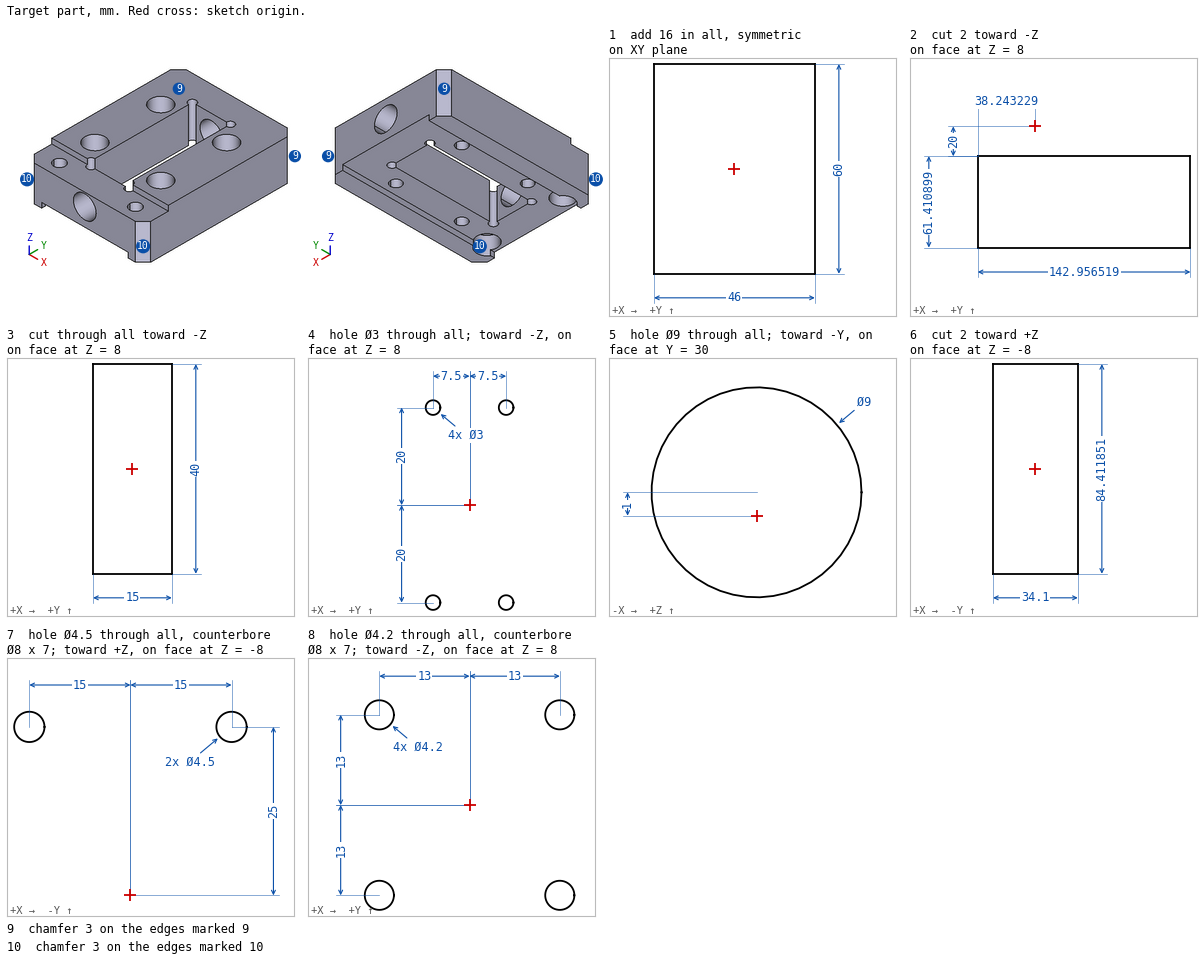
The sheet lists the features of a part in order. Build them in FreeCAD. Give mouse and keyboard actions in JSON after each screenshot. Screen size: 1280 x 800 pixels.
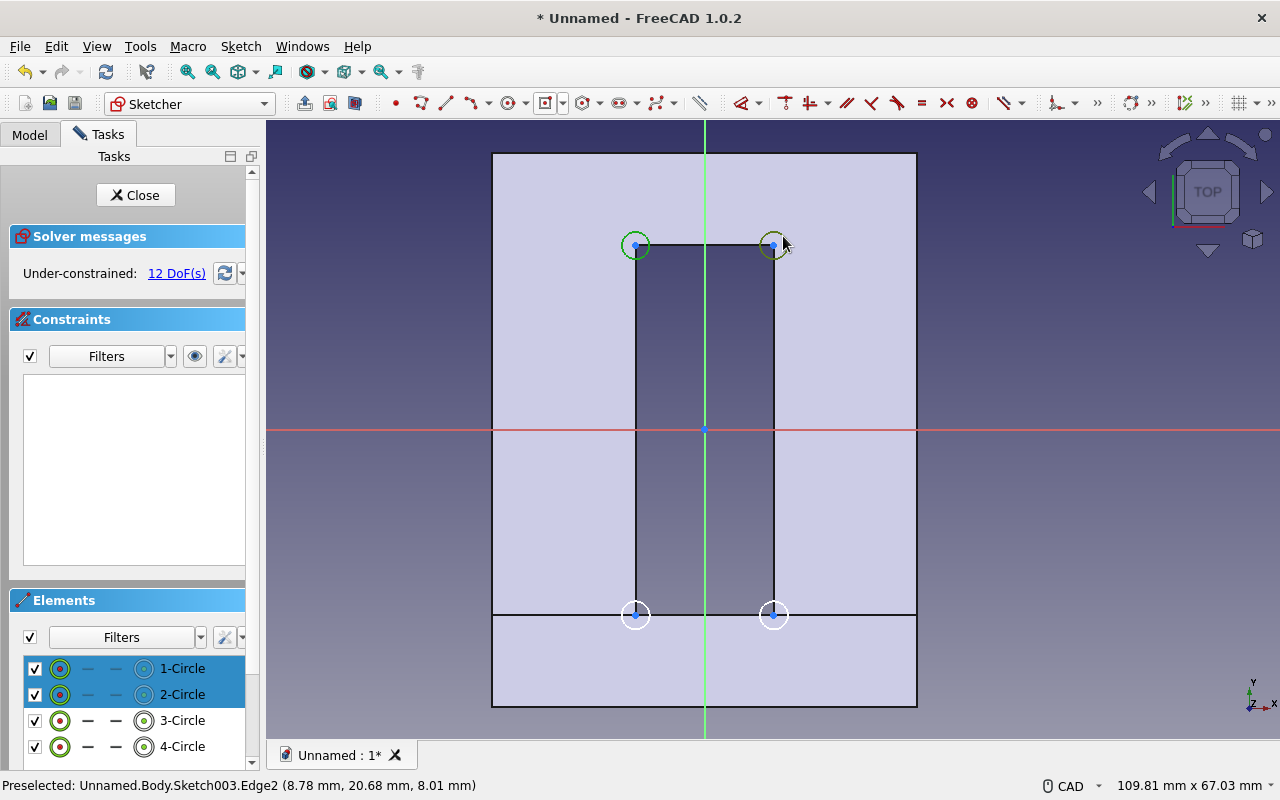
{"action": "left_click", "coordinate": [645, 605]}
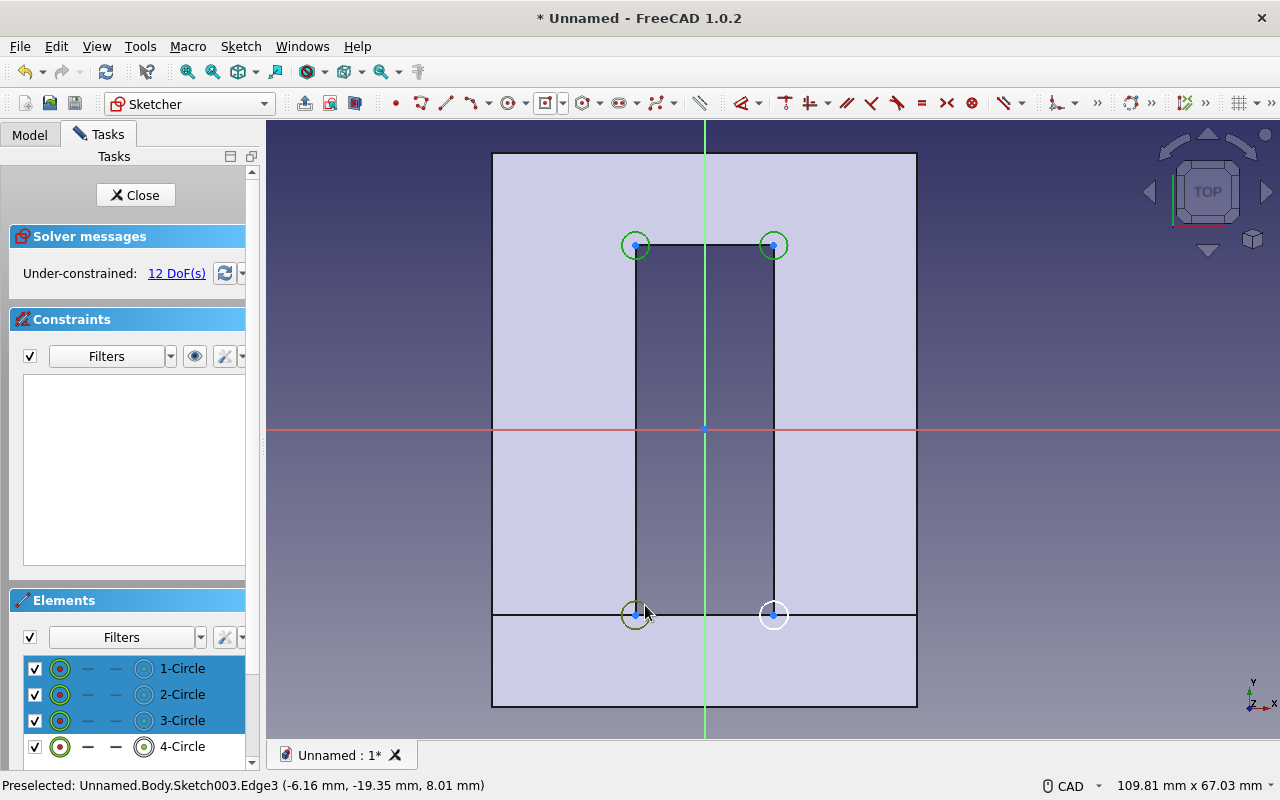
{"action": "left_click", "coordinate": [784, 605]}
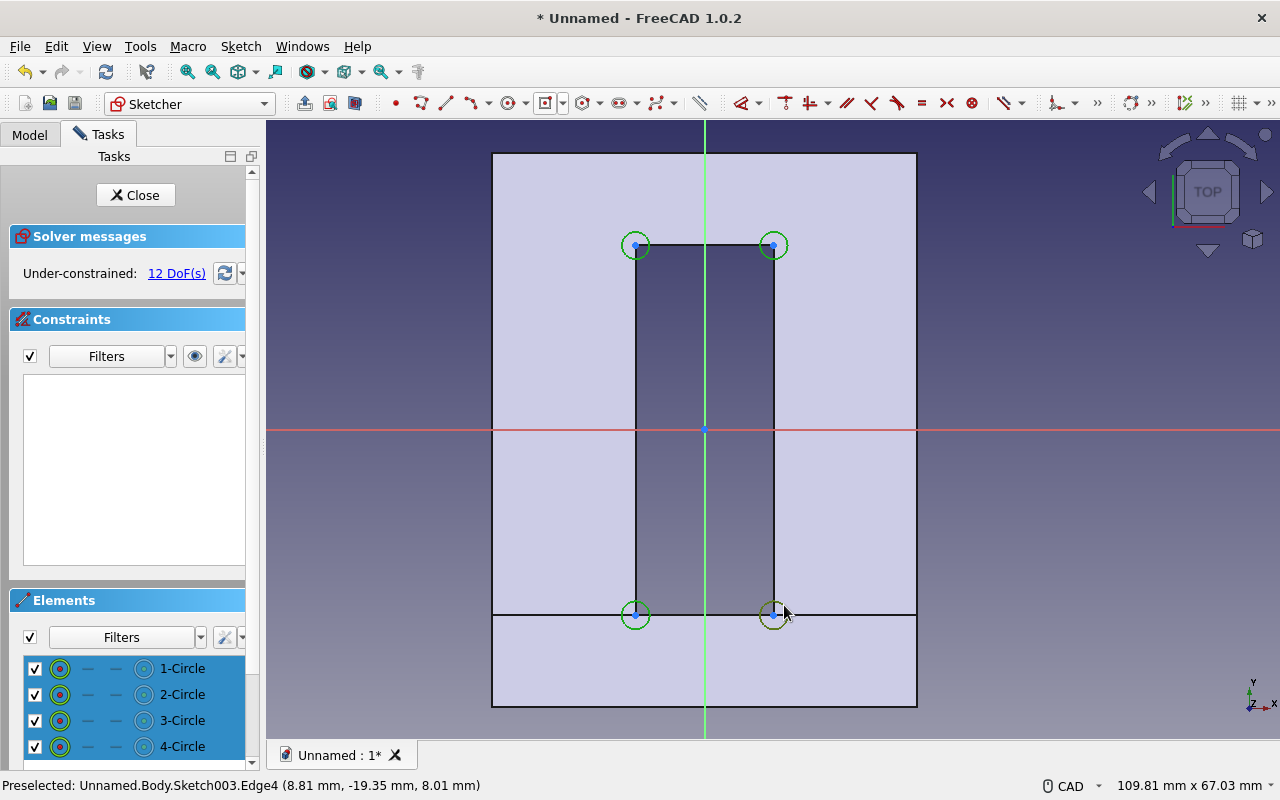
{"action": "left_click", "coordinate": [922, 104]}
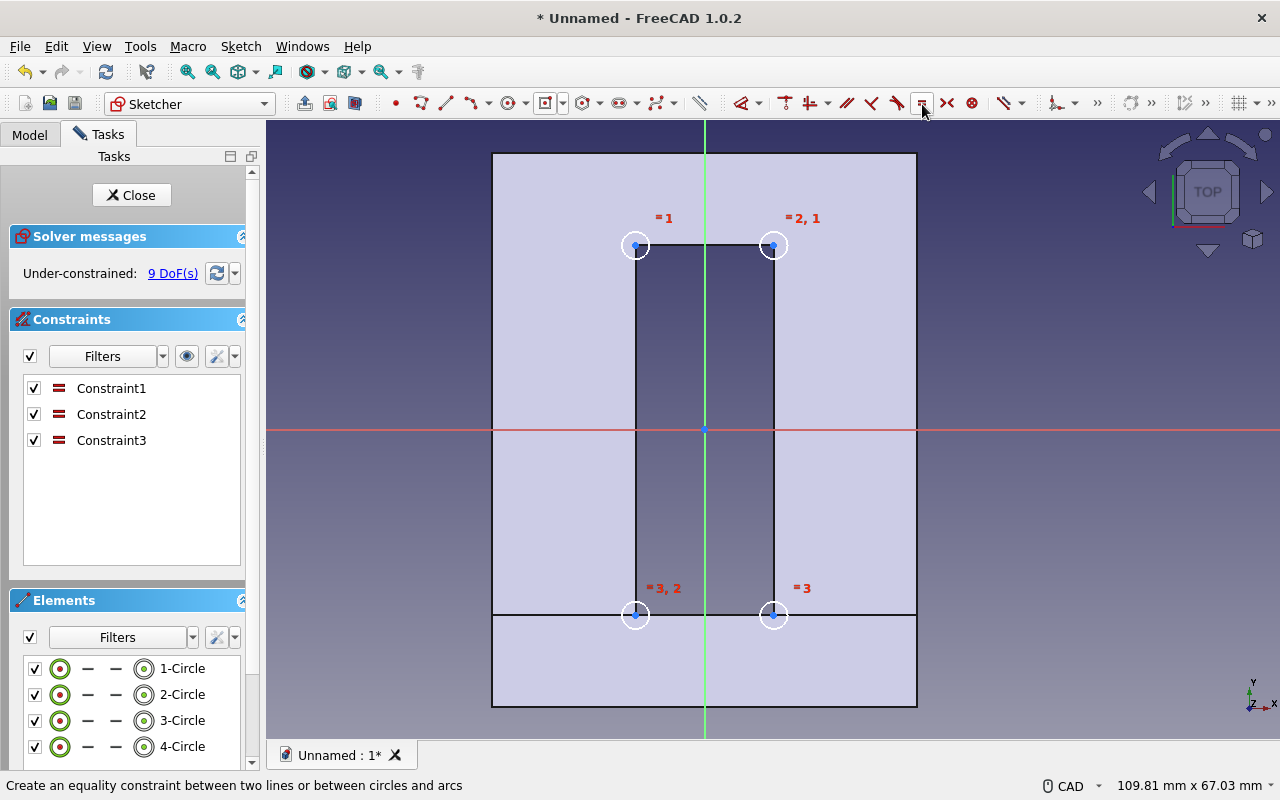
{"action": "left_click", "coordinate": [636, 246]}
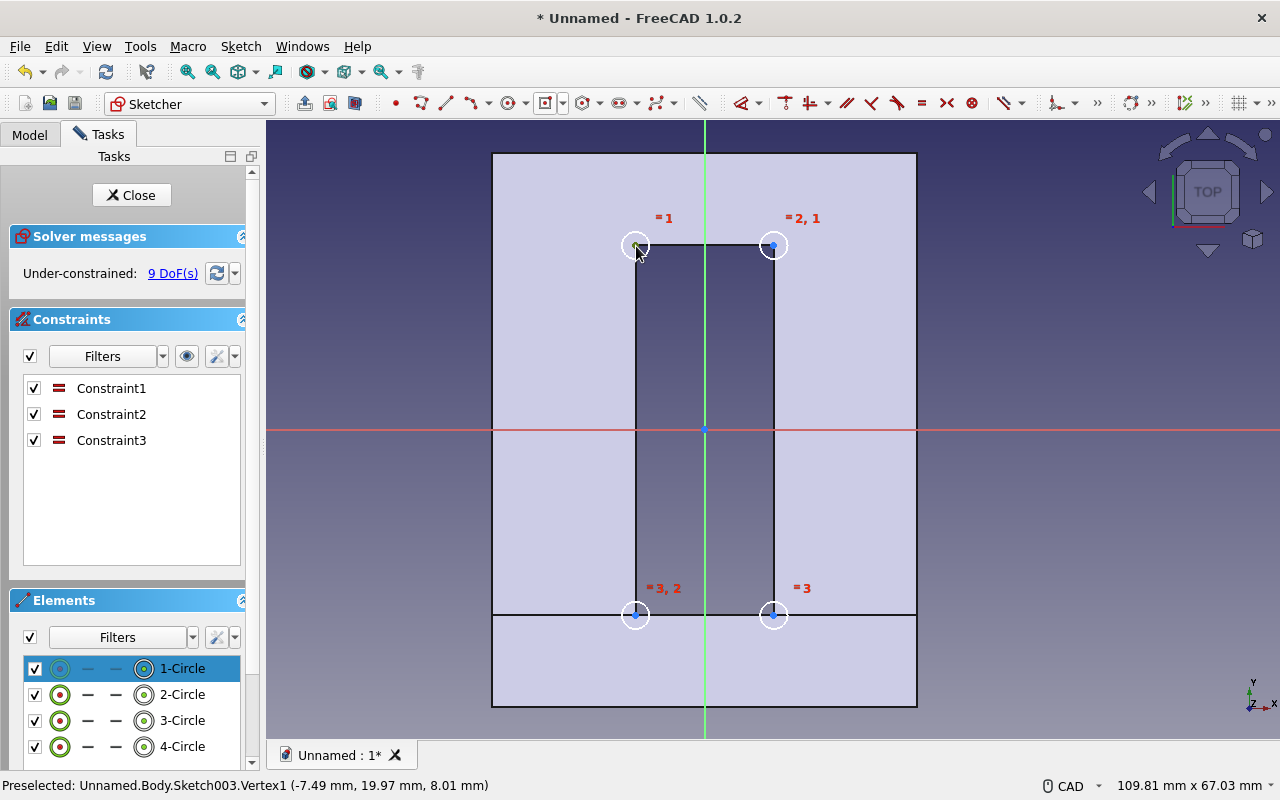
{"action": "left_click", "coordinate": [774, 246]}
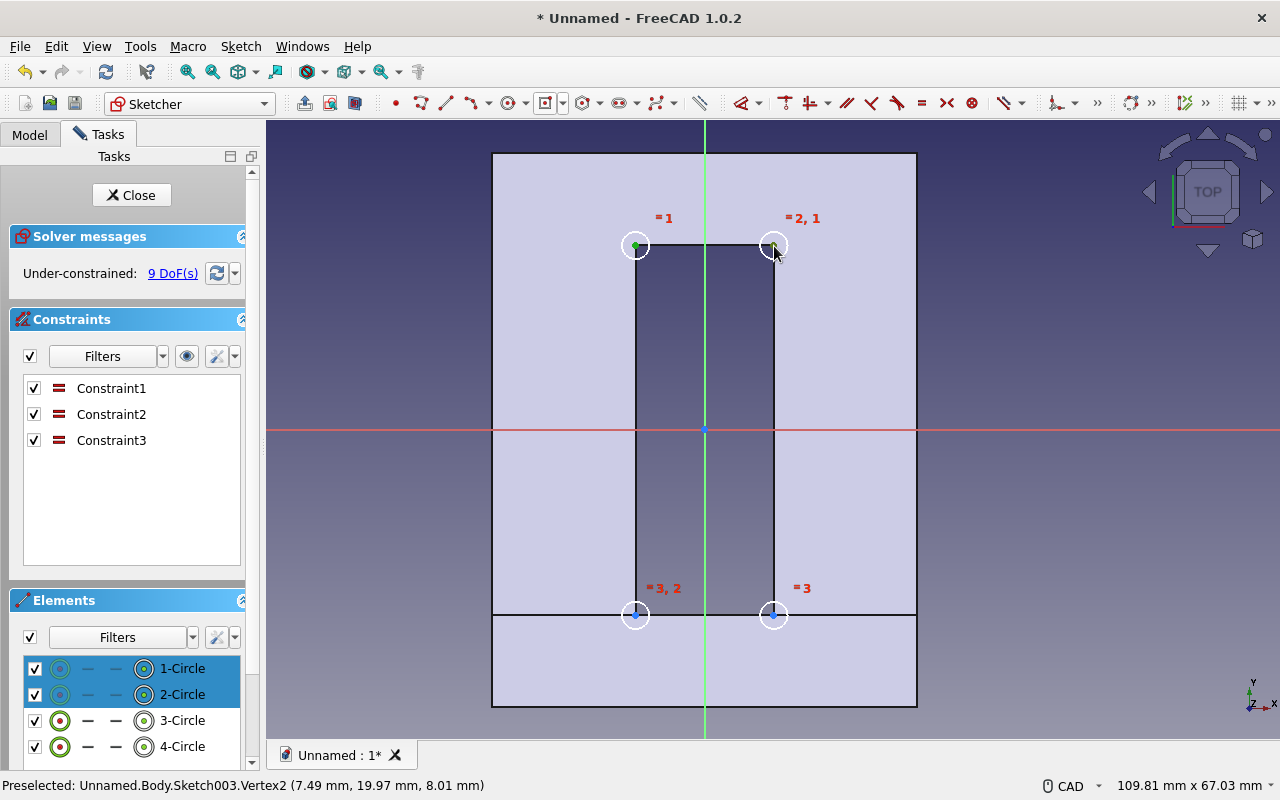
{"action": "left_click", "coordinate": [828, 104]}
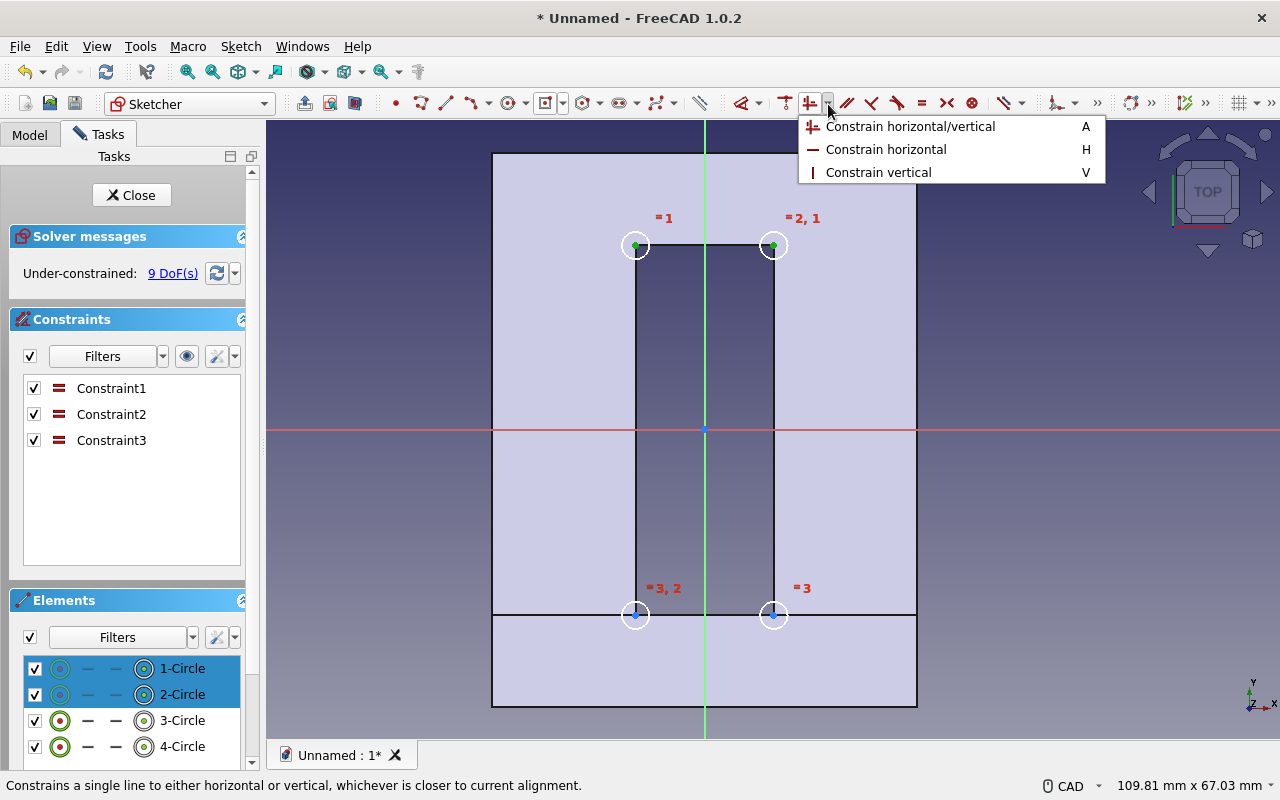
{"action": "left_click", "coordinate": [952, 150]}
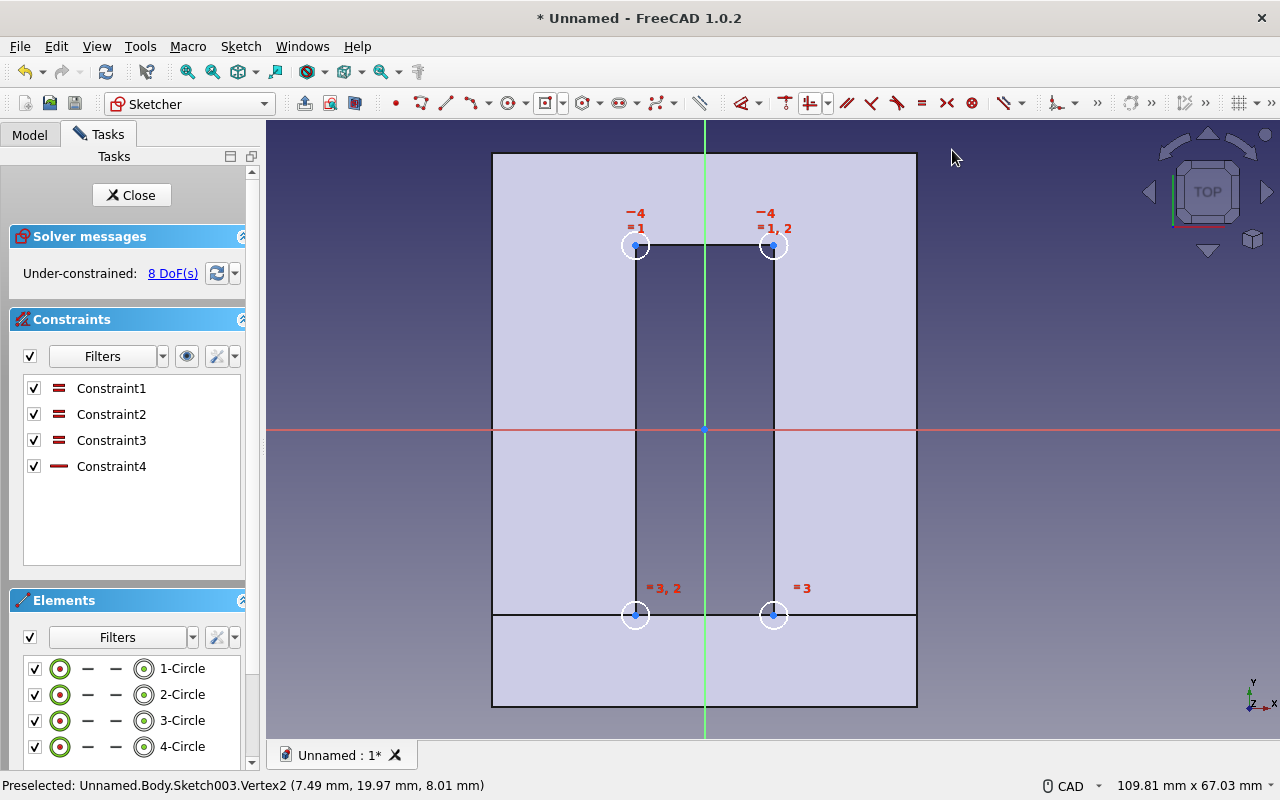
{"action": "left_click", "coordinate": [636, 246]}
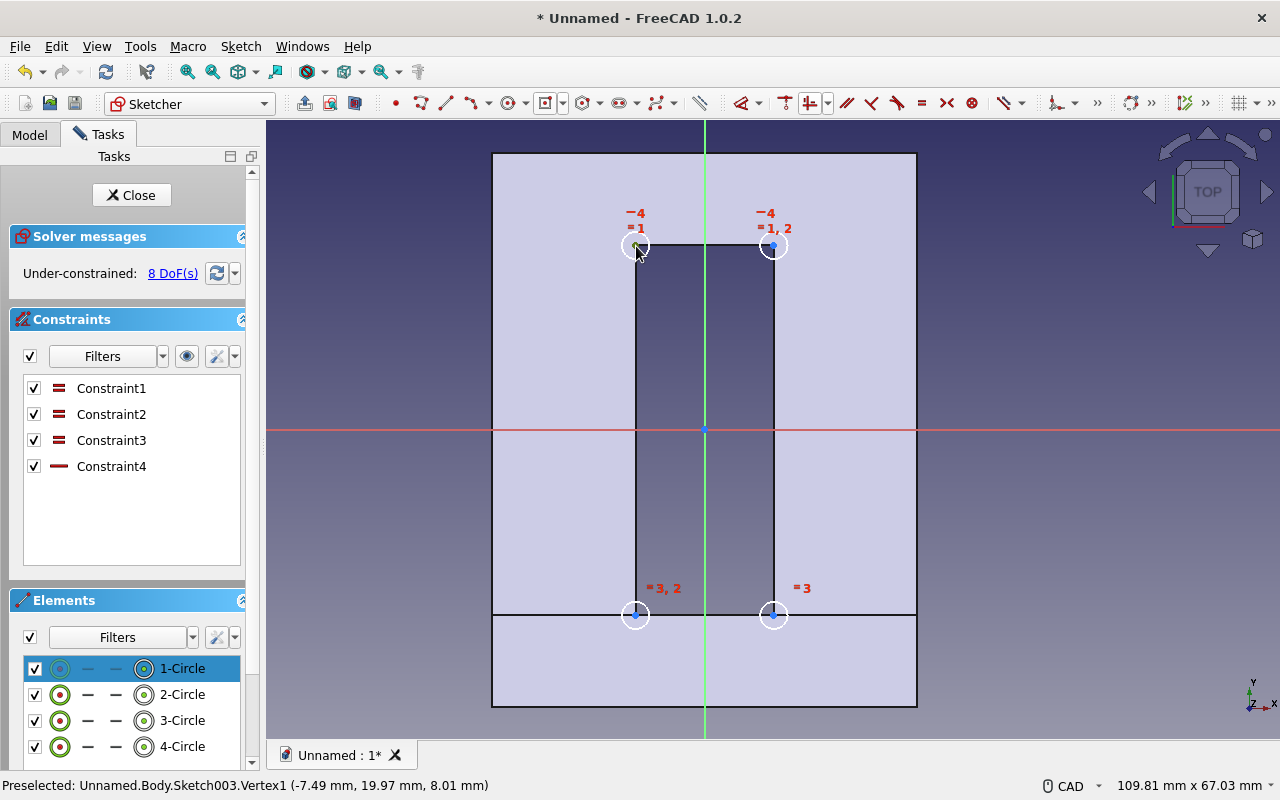
{"action": "left_click", "coordinate": [636, 615]}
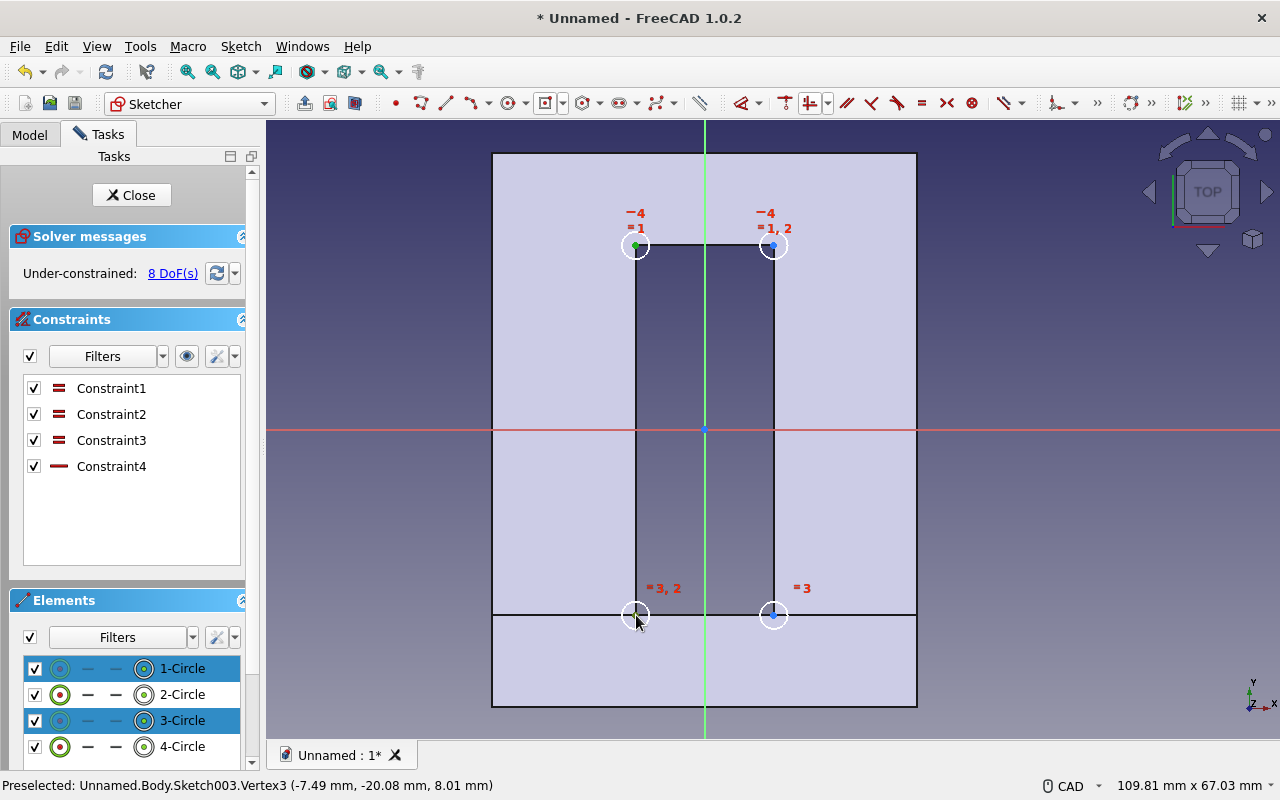
{"action": "key", "text": "v"}